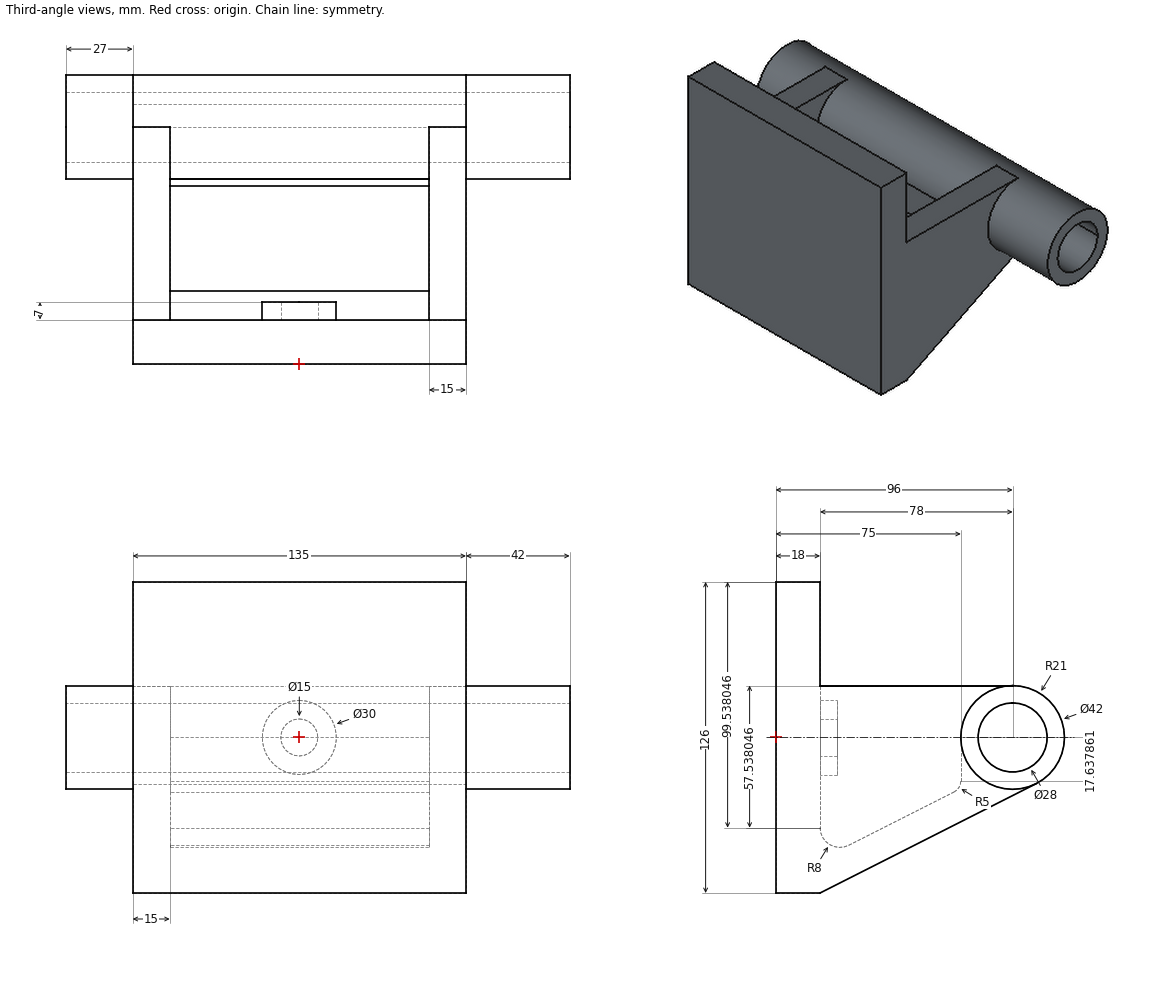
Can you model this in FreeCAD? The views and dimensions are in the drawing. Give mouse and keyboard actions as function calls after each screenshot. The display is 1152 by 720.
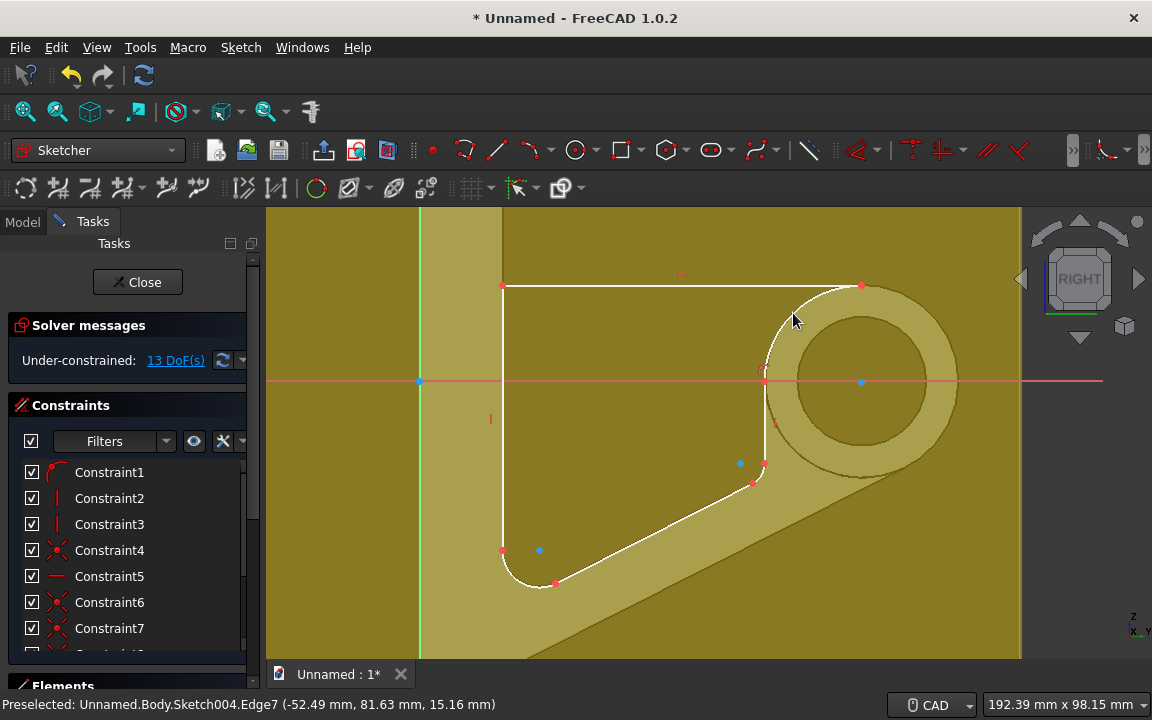
click(765, 406)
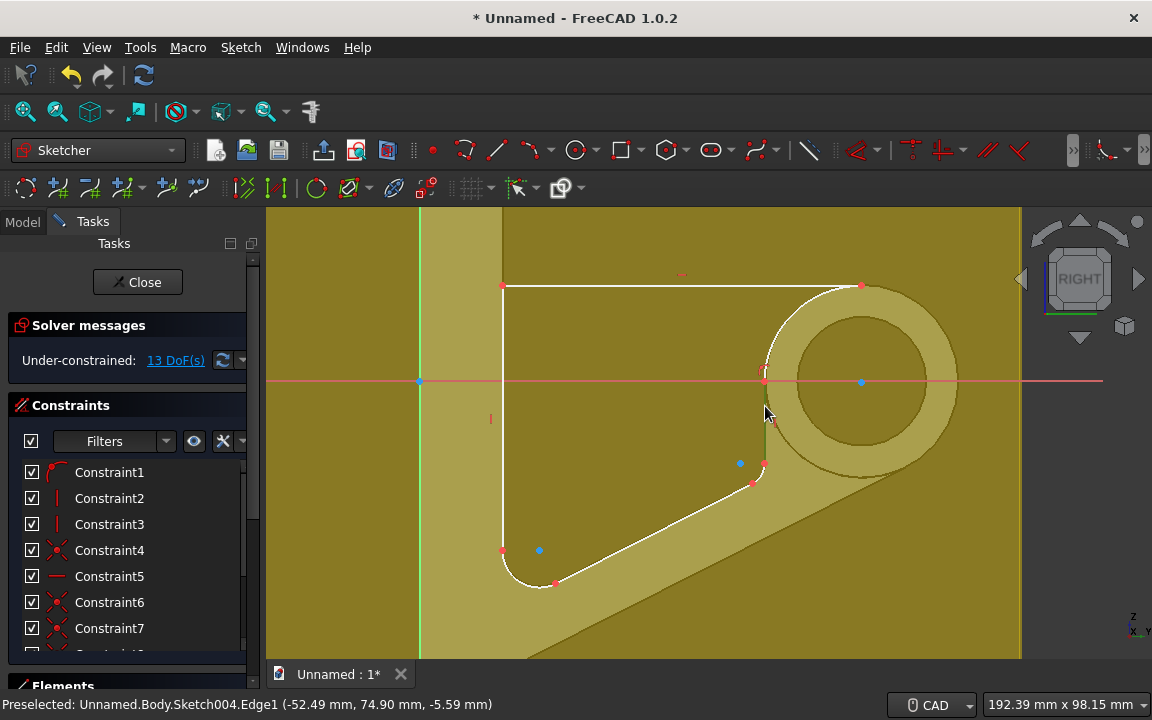
click(761, 475)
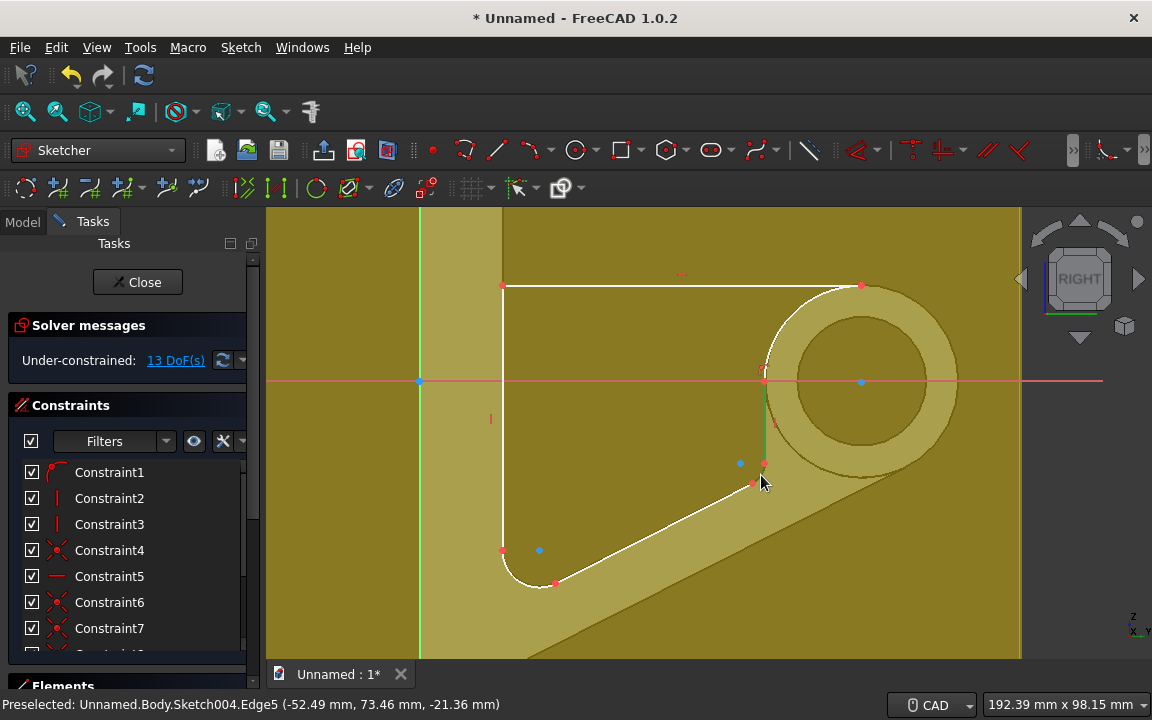
key(t)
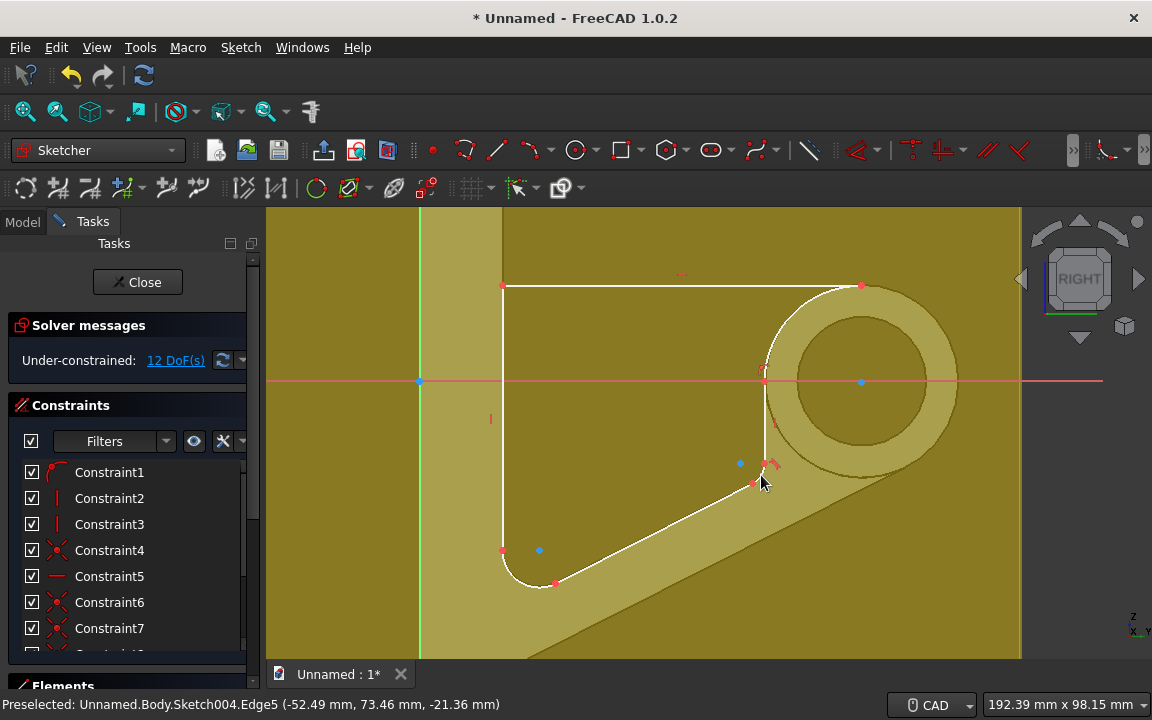
click(765, 406)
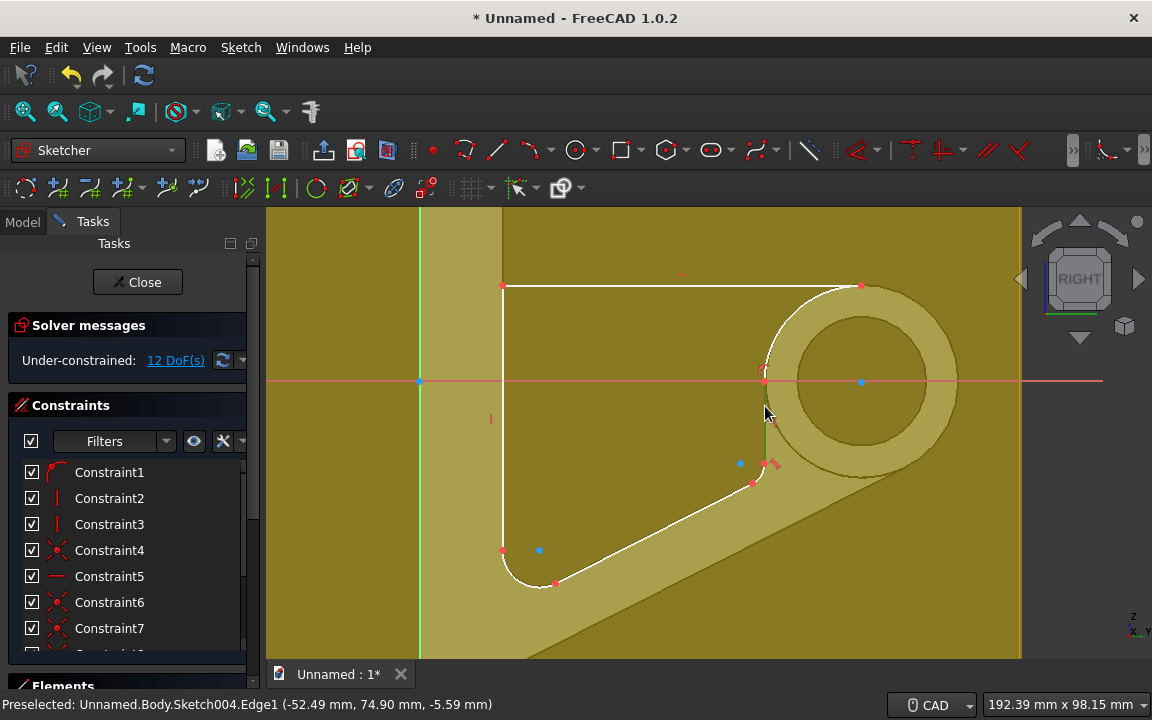
scroll(818, 296, up, 2)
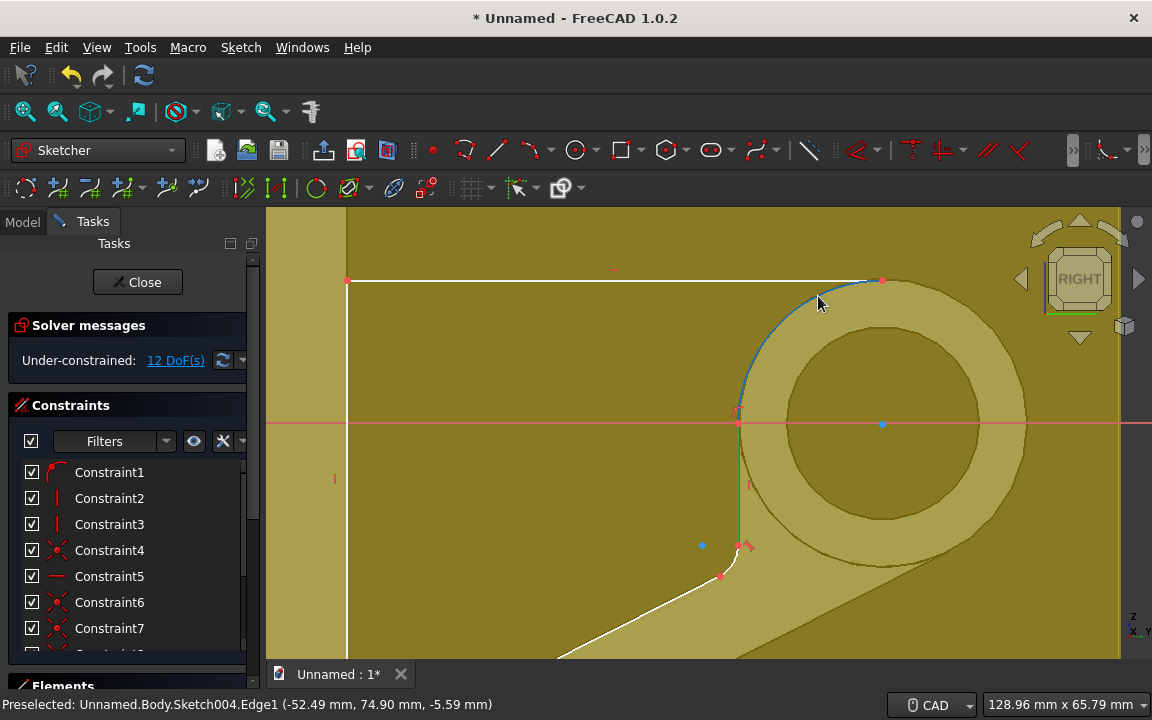
click(818, 296)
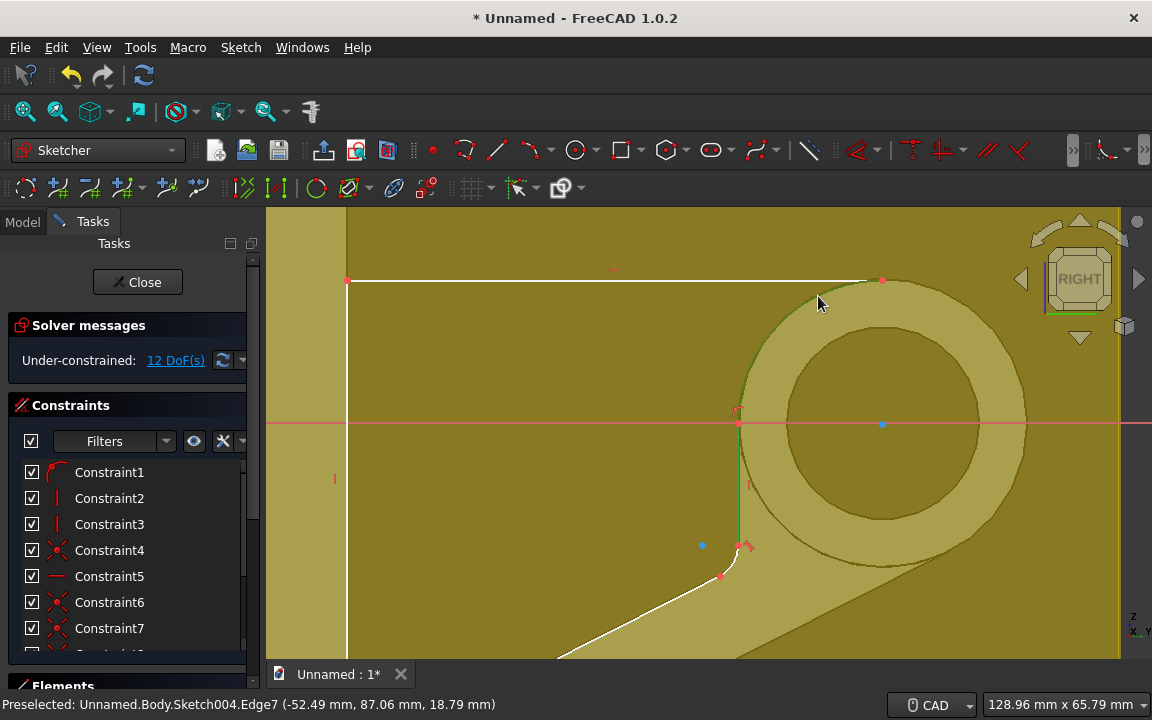
key(t)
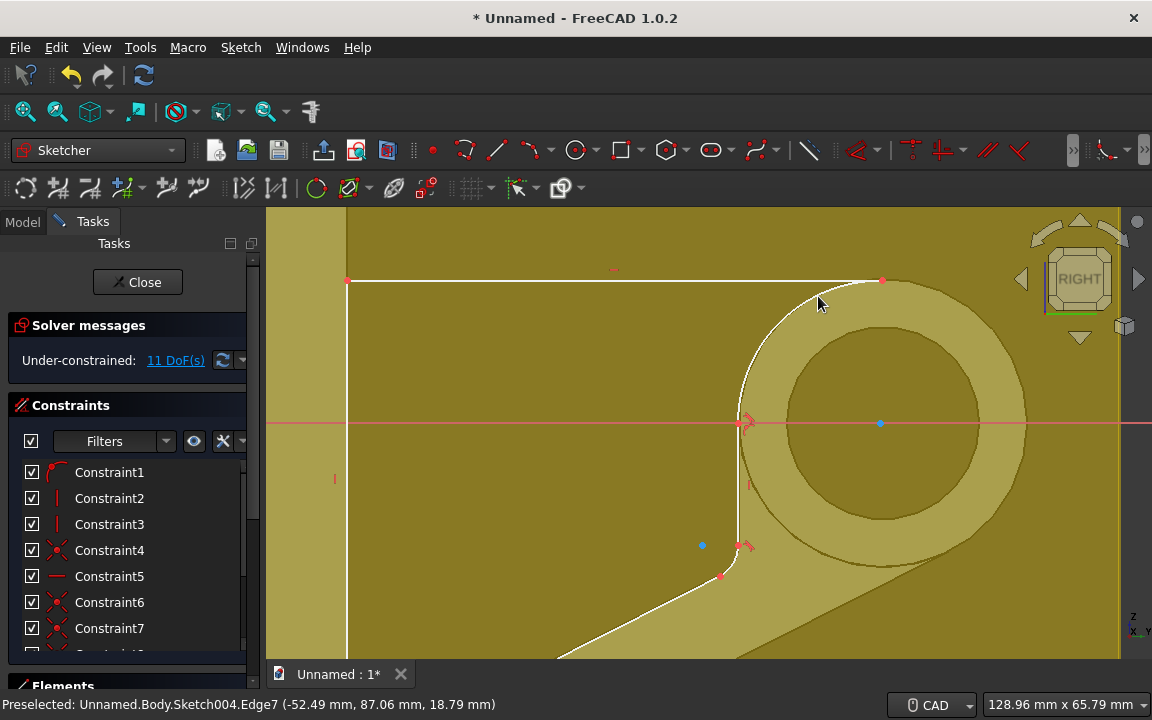
click(632, 621)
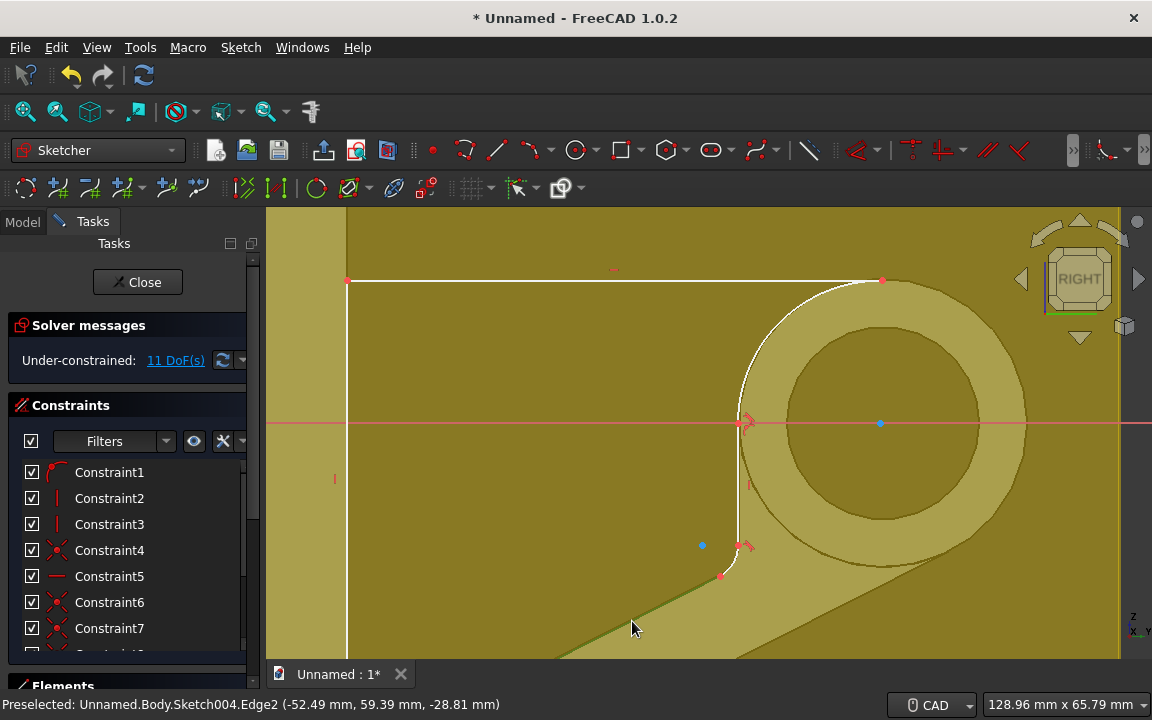
scroll(729, 569, up, 2)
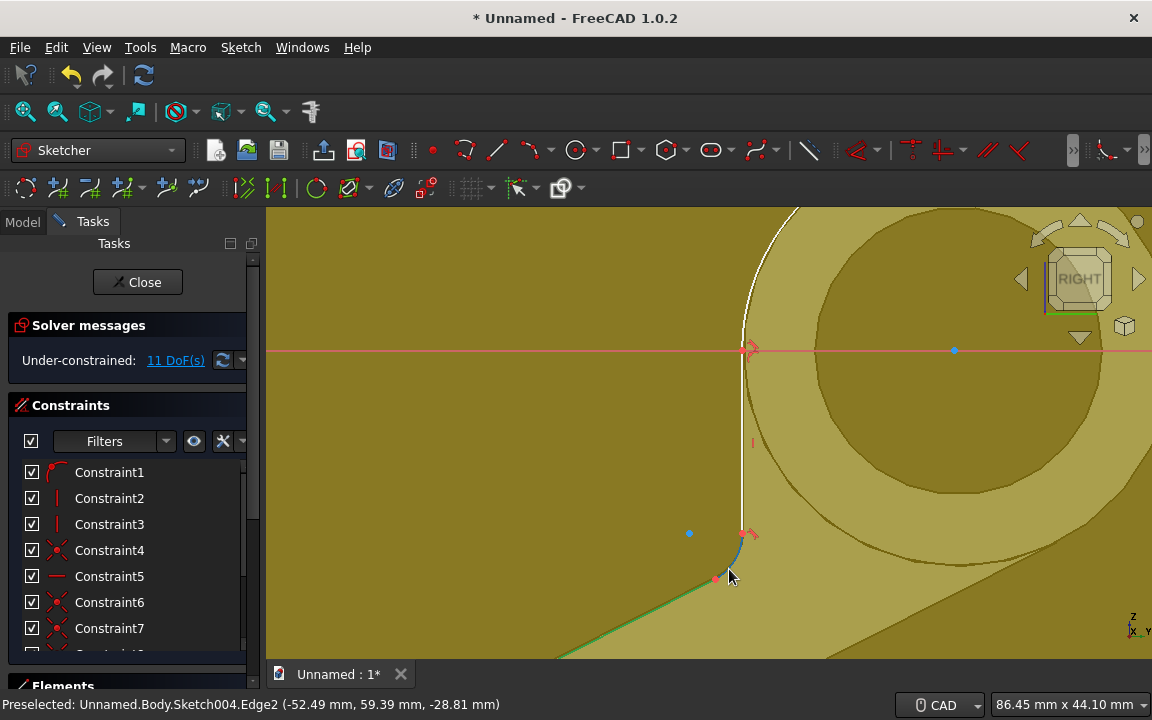
click(728, 569)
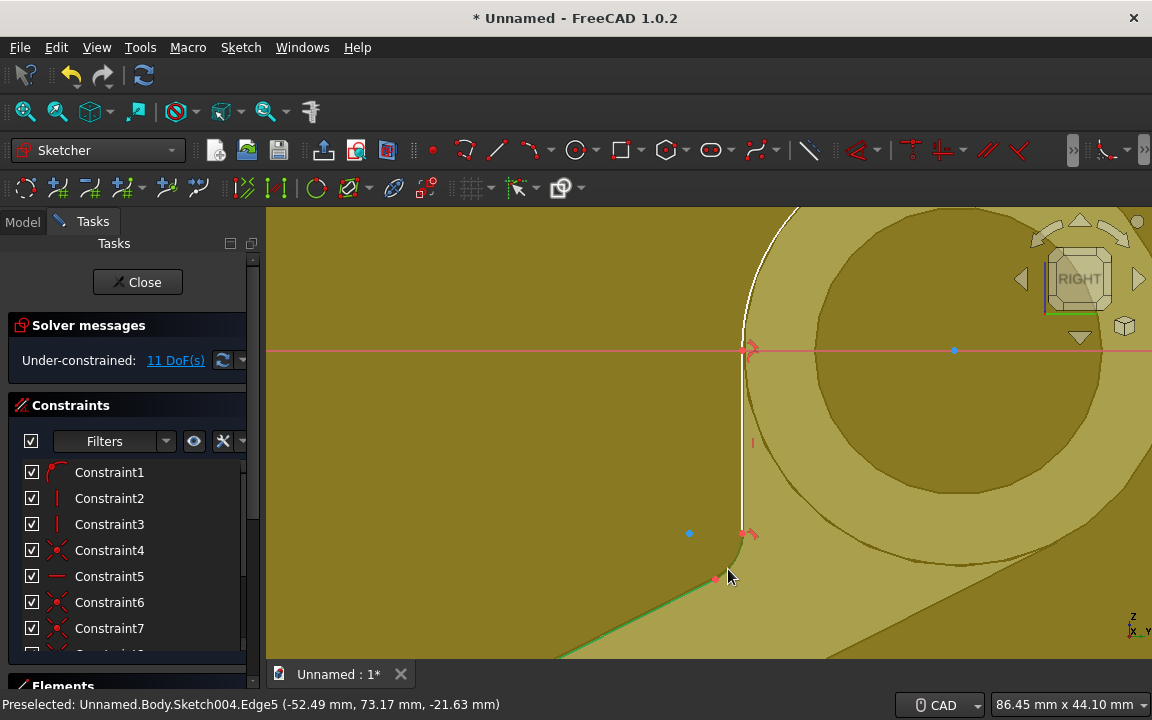
key(t)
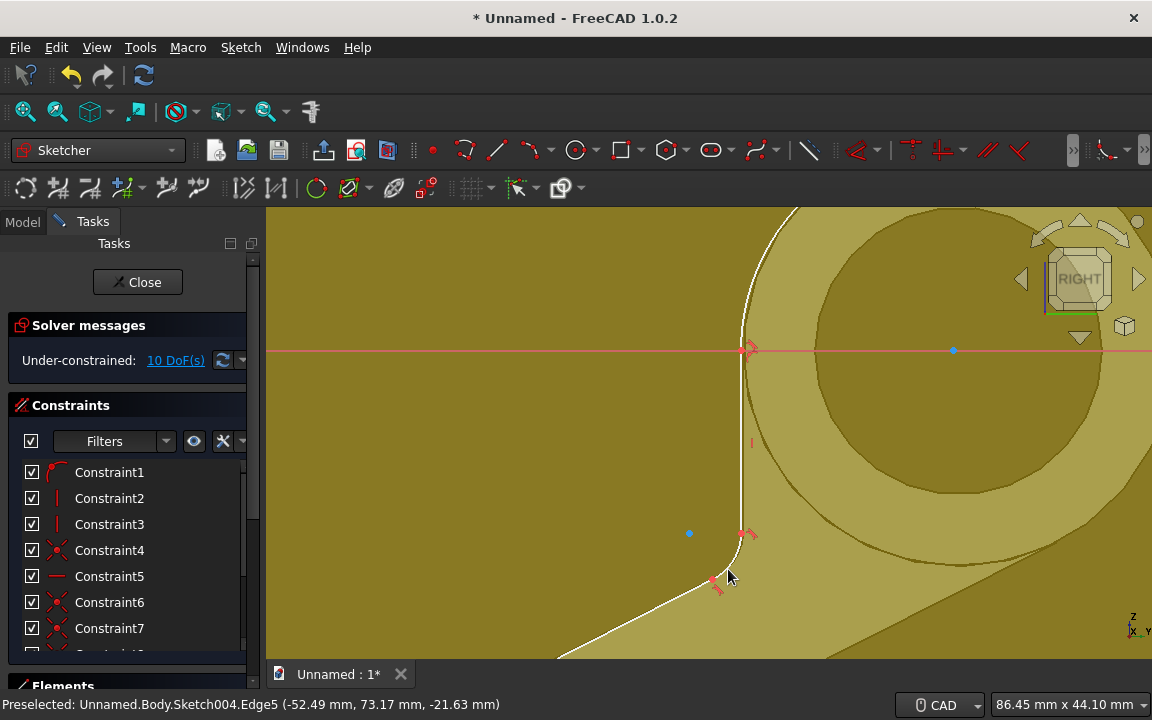
click(626, 624)